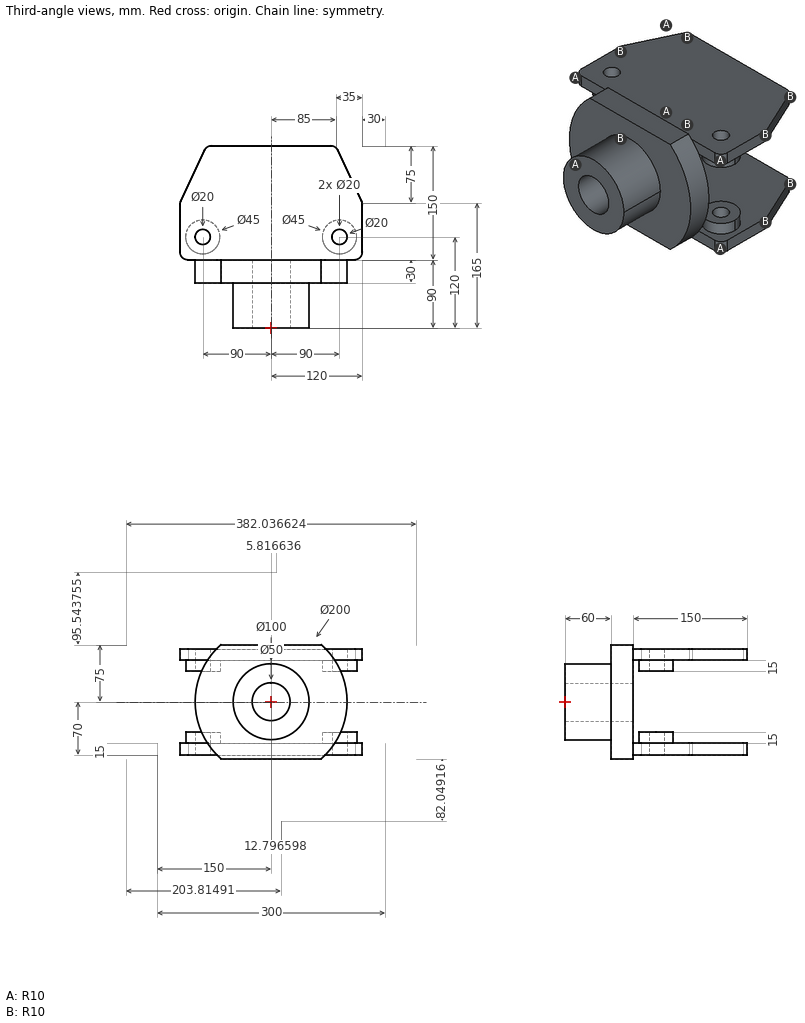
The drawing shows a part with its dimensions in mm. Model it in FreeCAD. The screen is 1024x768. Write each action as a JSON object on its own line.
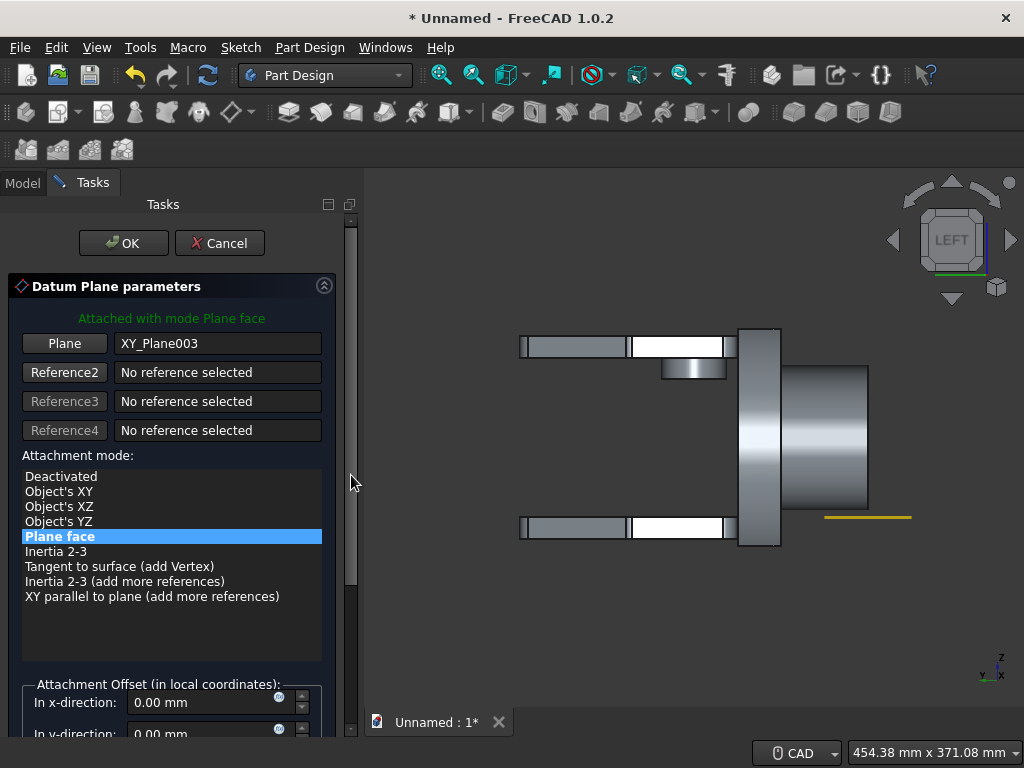
{"action": "left_click", "coordinate": [124, 243]}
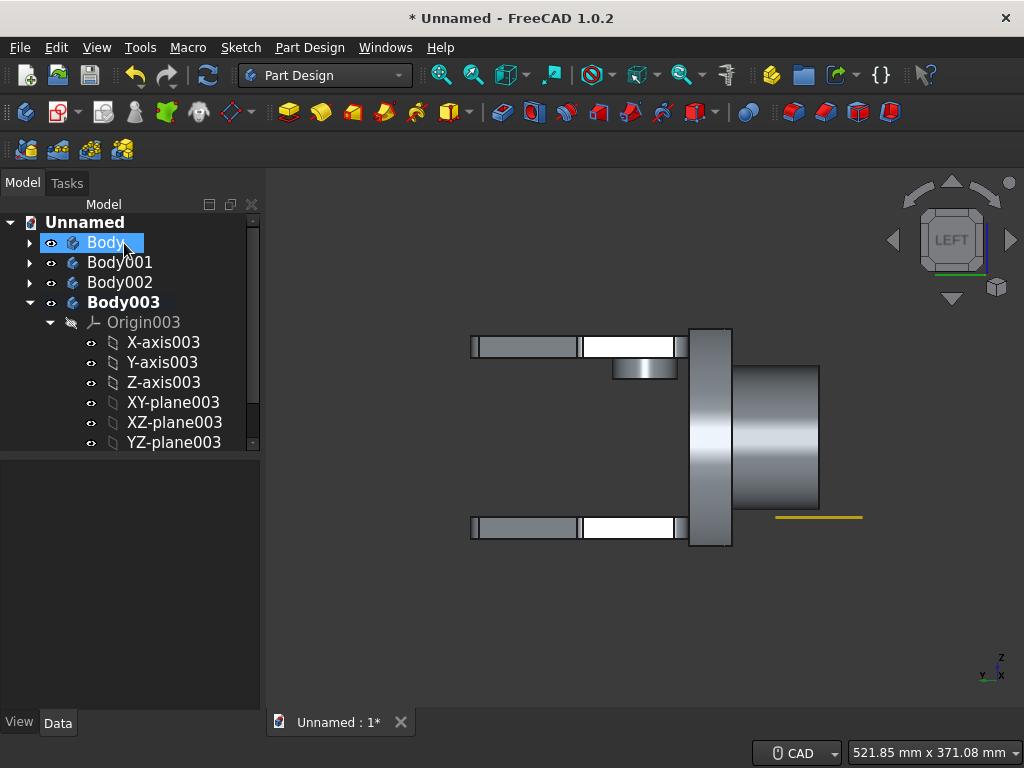
{"action": "scroll", "coordinate": [100, 338], "scroll_direction": "down", "scroll_amount": 3}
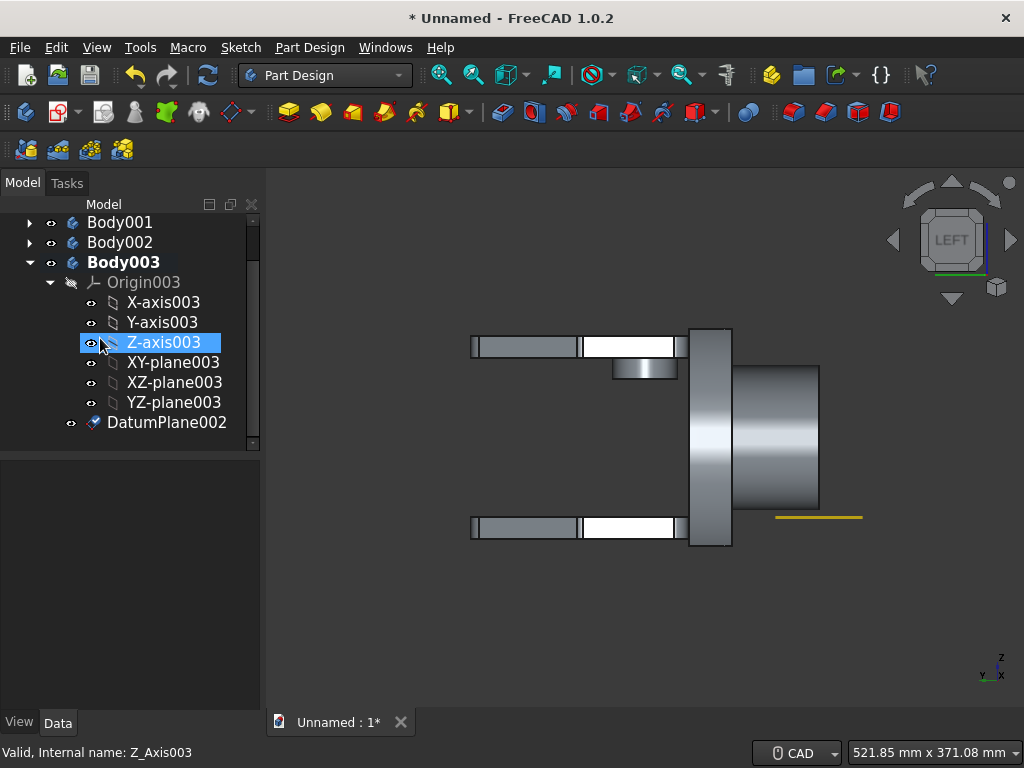
{"action": "left_click", "coordinate": [116, 423]}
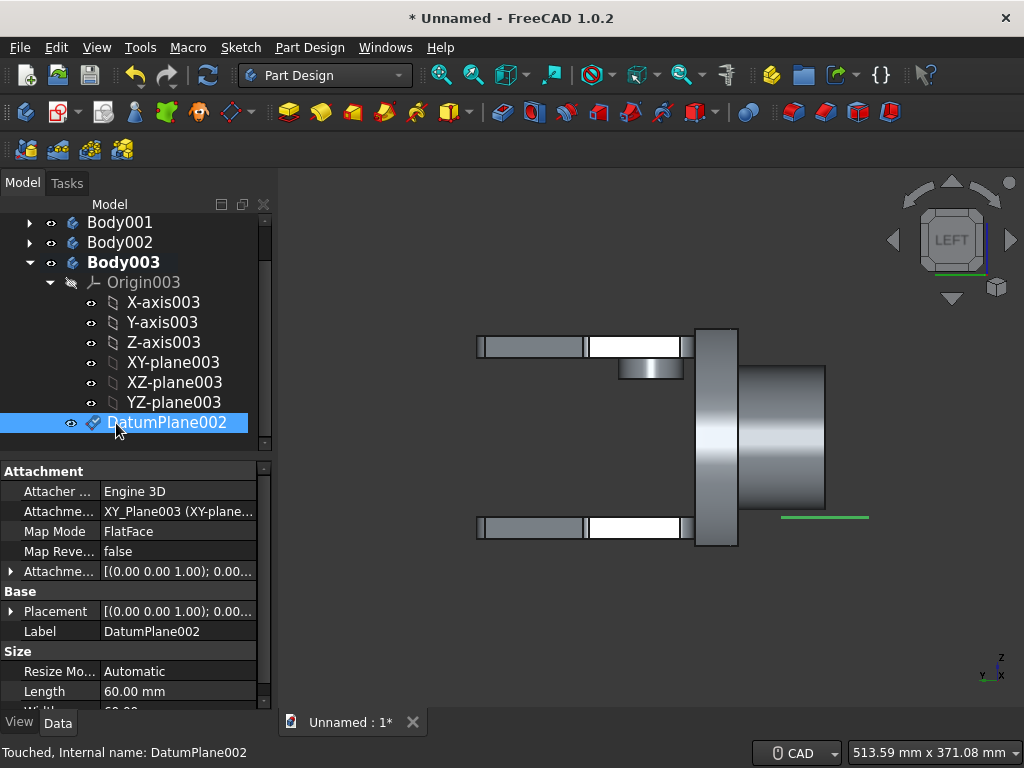
{"action": "left_click", "coordinate": [58, 112]}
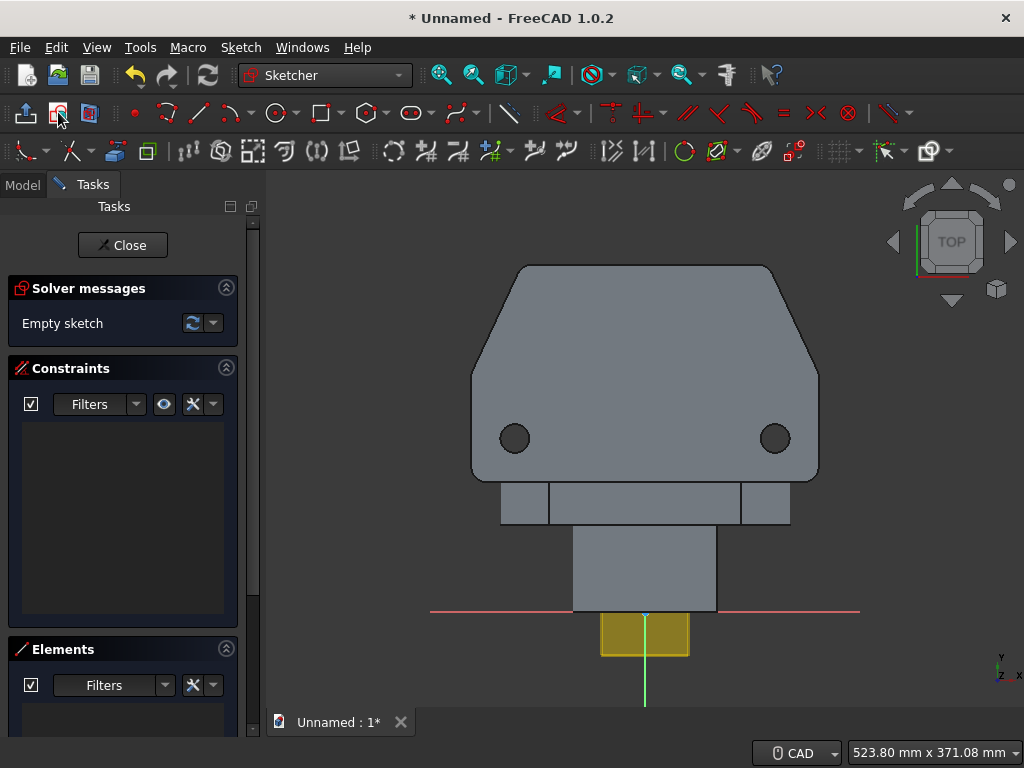
{"action": "scroll", "coordinate": [826, 439], "scroll_direction": "up", "scroll_amount": 8}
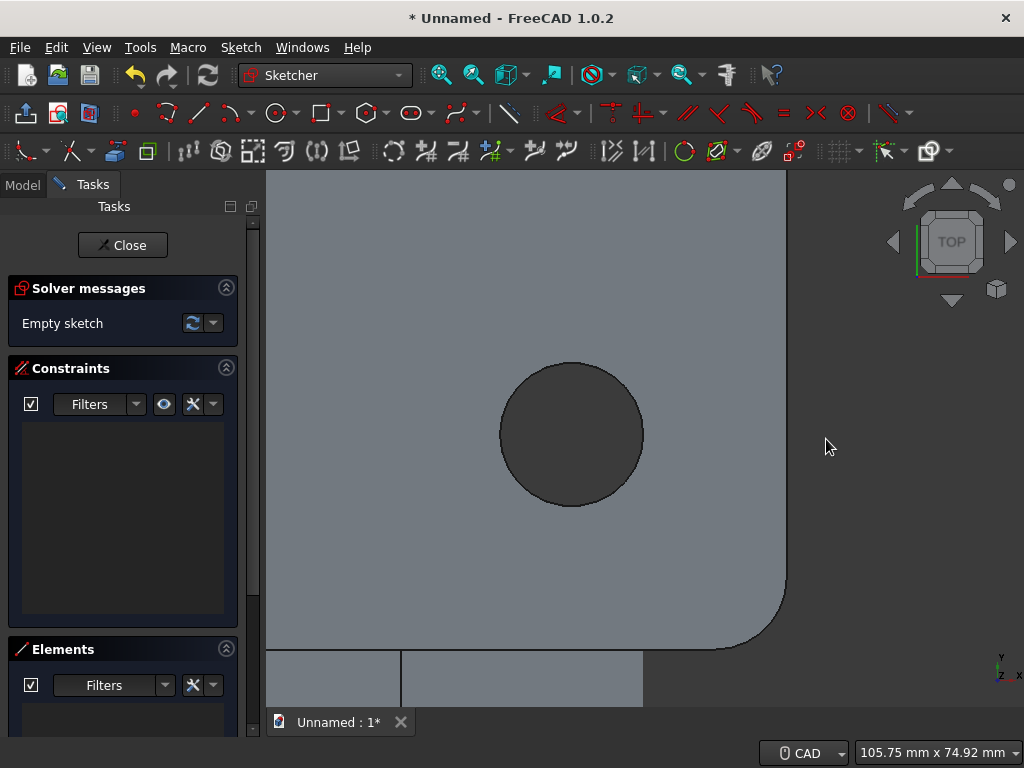
{"action": "left_click", "coordinate": [276, 114]}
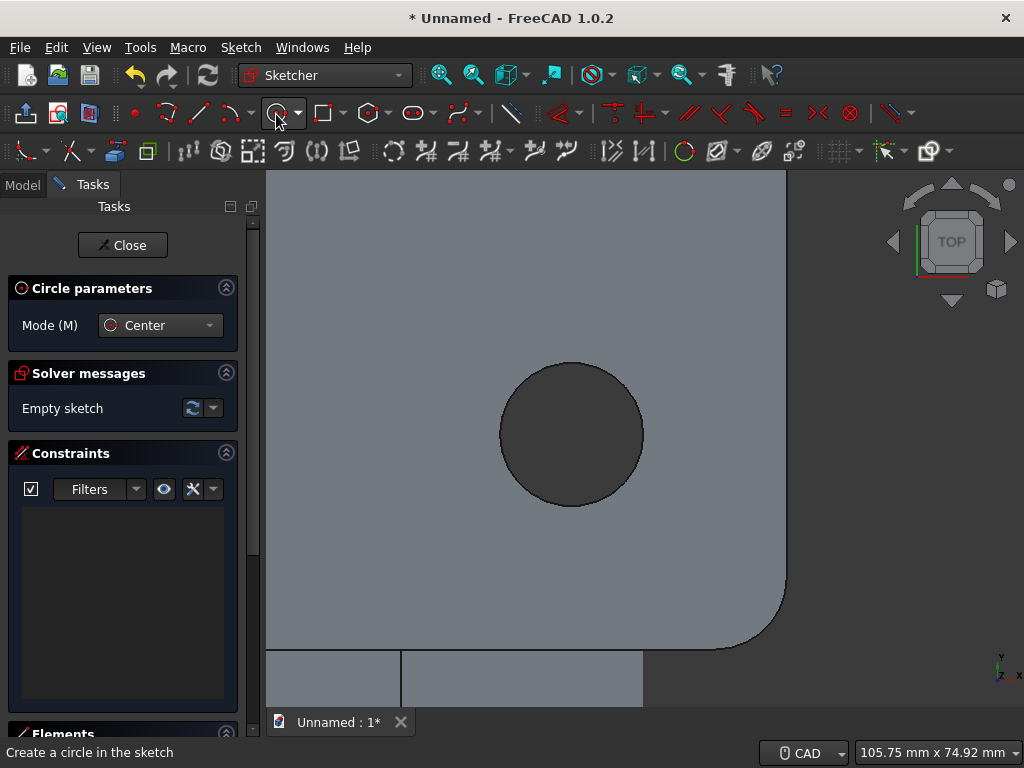
{"action": "left_click", "coordinate": [572, 435]}
{"action": "left_click", "coordinate": [686, 321]}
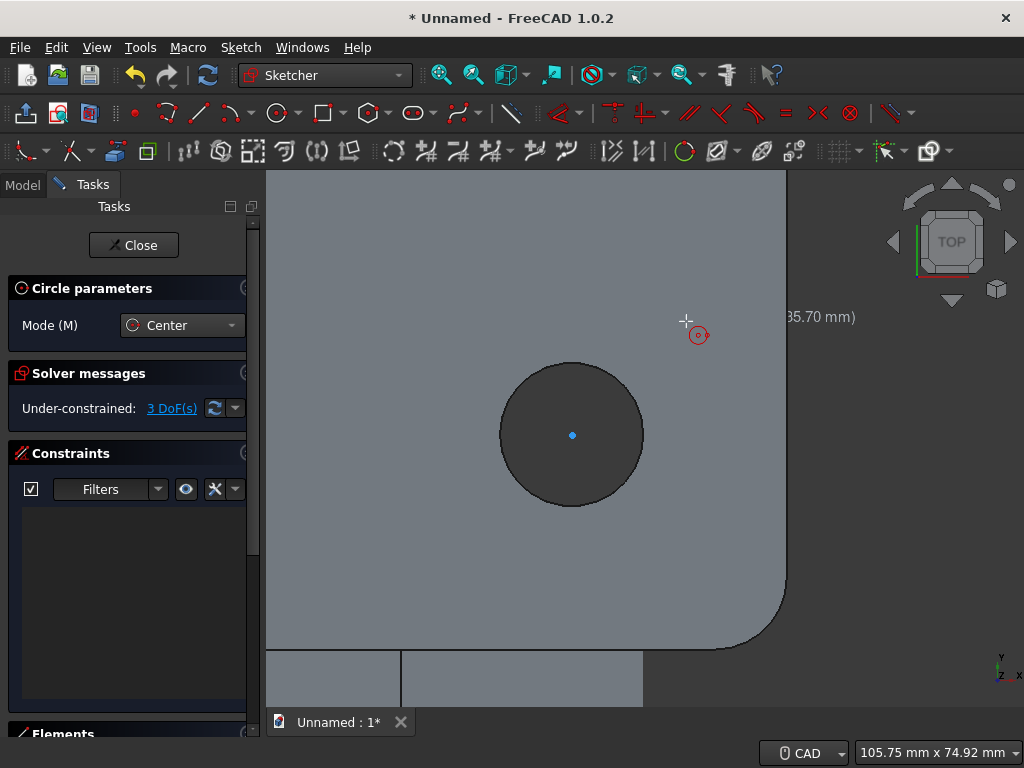
{"action": "left_click", "coordinate": [572, 436]}
{"action": "left_click", "coordinate": [622, 384]}
{"action": "key", "text": "Escape"}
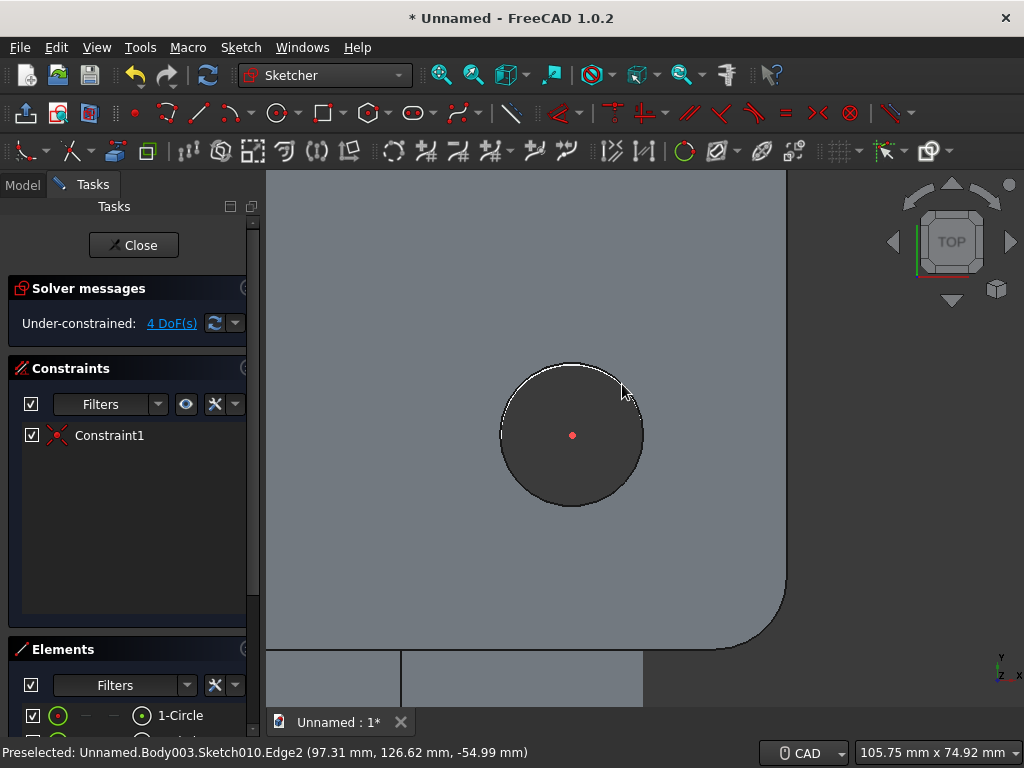
{"action": "key", "text": "d"}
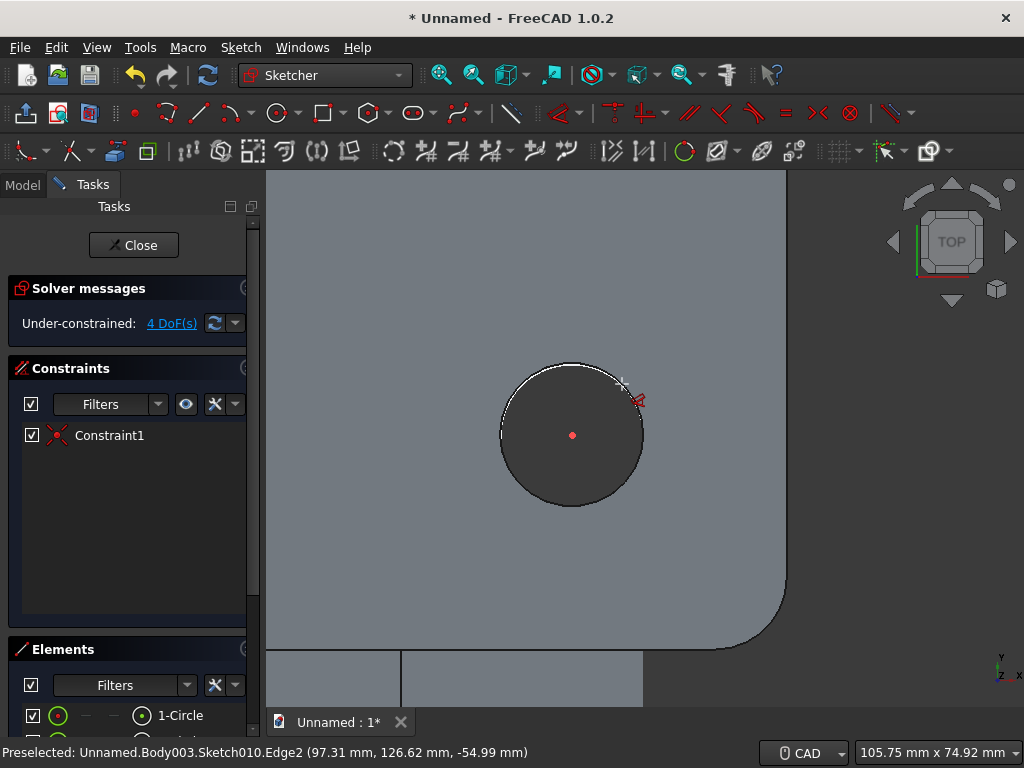
{"action": "left_click", "coordinate": [686, 322]}
{"action": "left_click", "coordinate": [709, 299]}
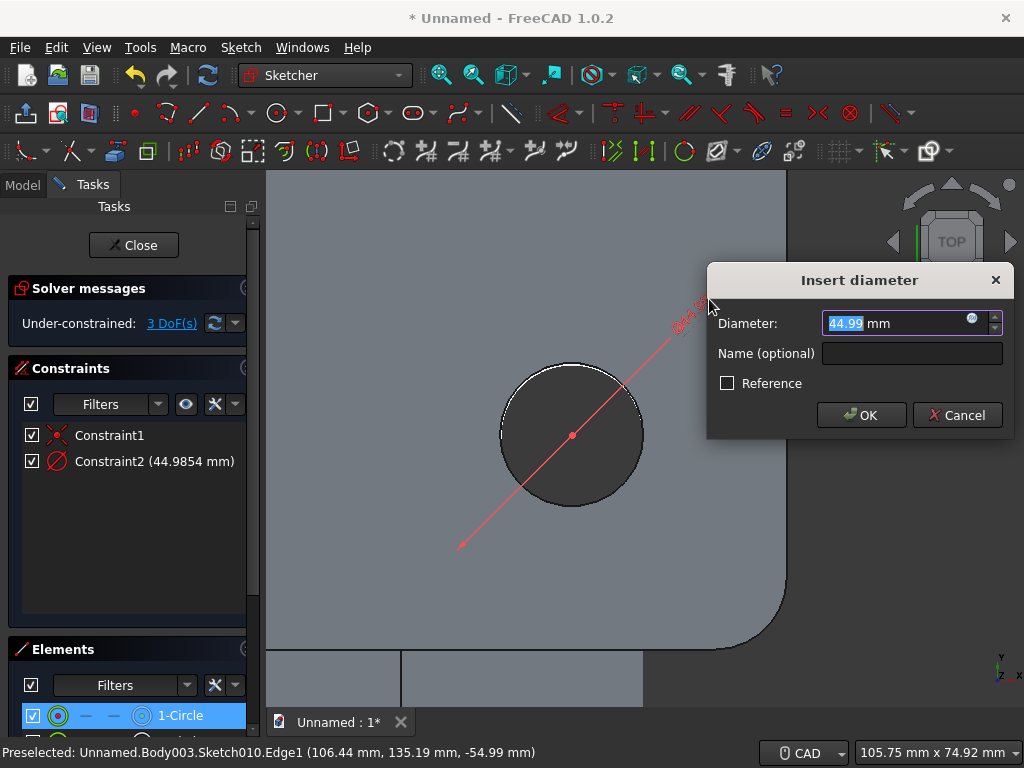
{"action": "type", "text": "45"}
{"action": "key", "text": "Return"}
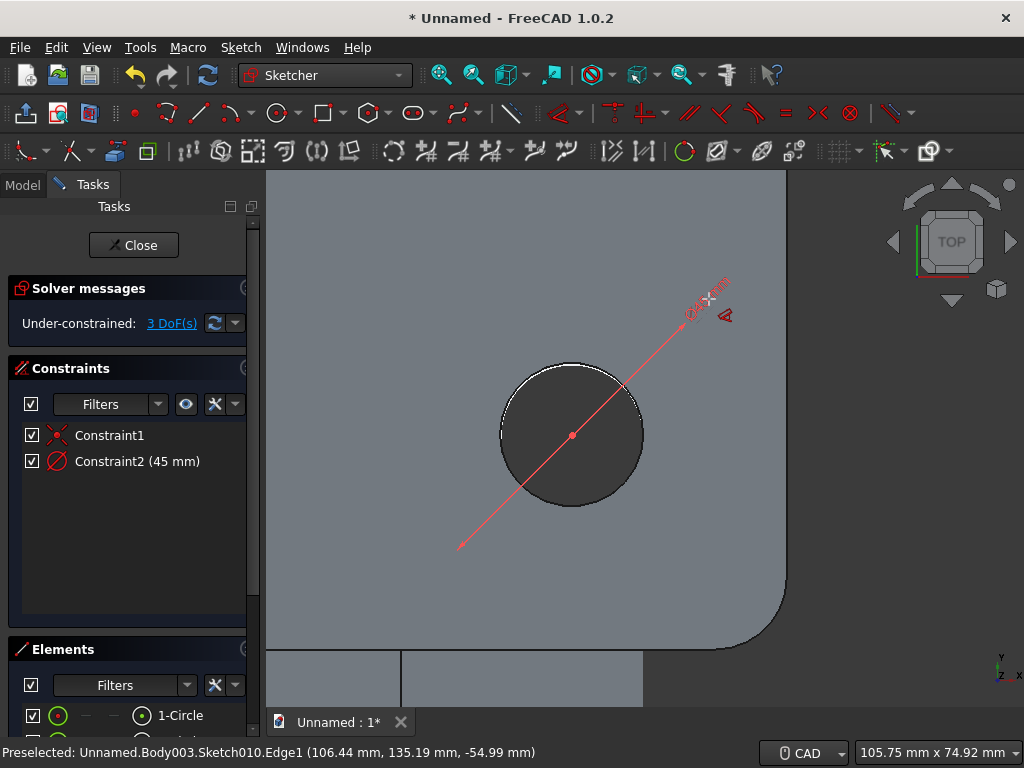
{"action": "left_click", "coordinate": [622, 385]}
{"action": "left_click", "coordinate": [644, 362]}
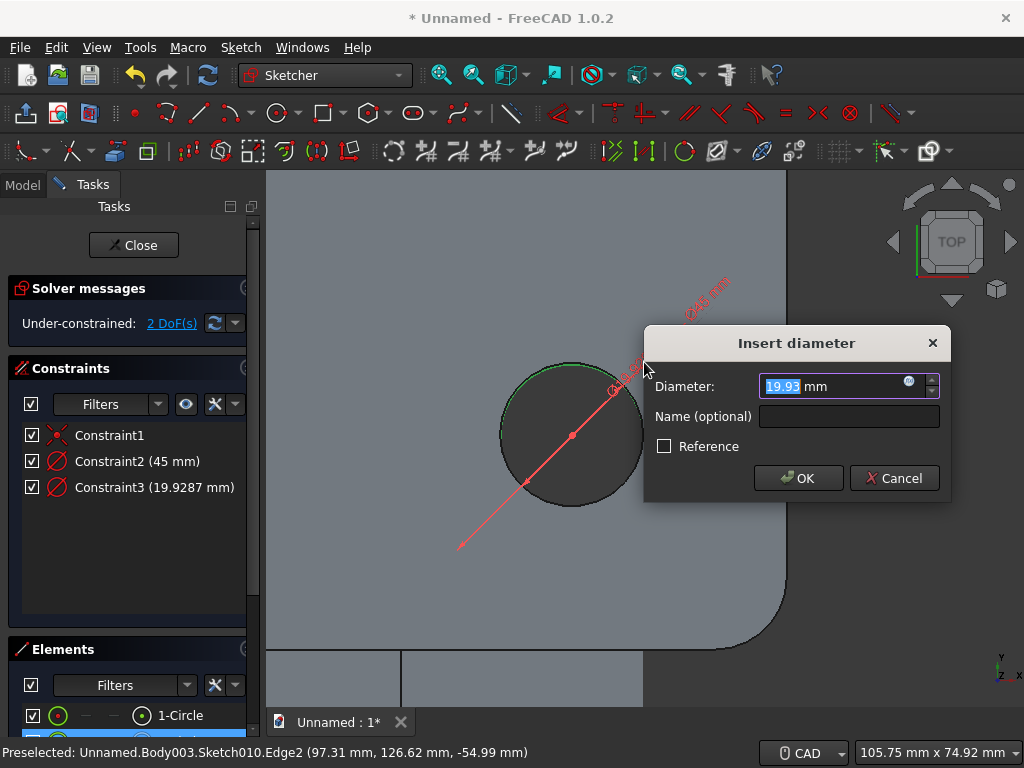
{"action": "type", "text": "20"}
{"action": "key", "text": "Return"}